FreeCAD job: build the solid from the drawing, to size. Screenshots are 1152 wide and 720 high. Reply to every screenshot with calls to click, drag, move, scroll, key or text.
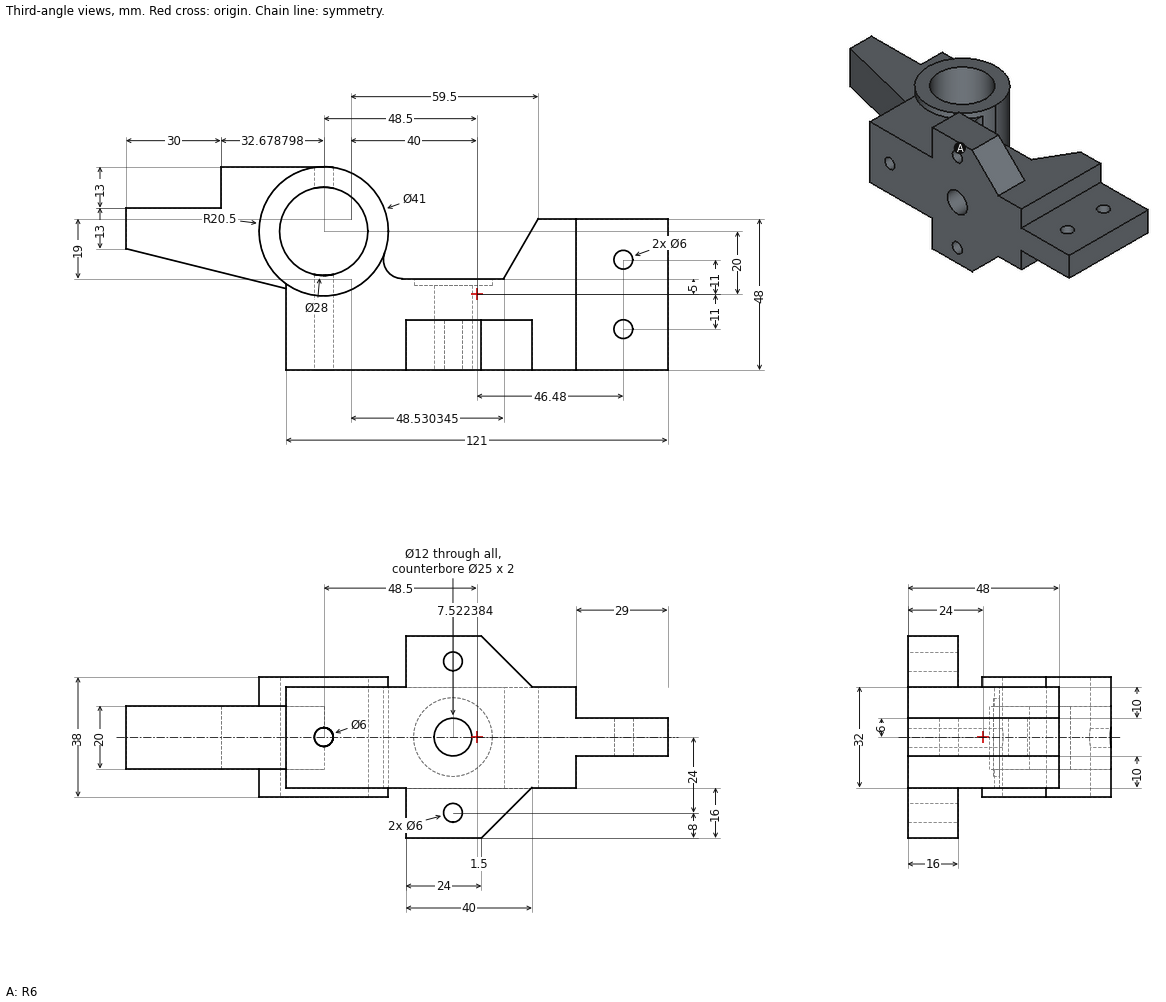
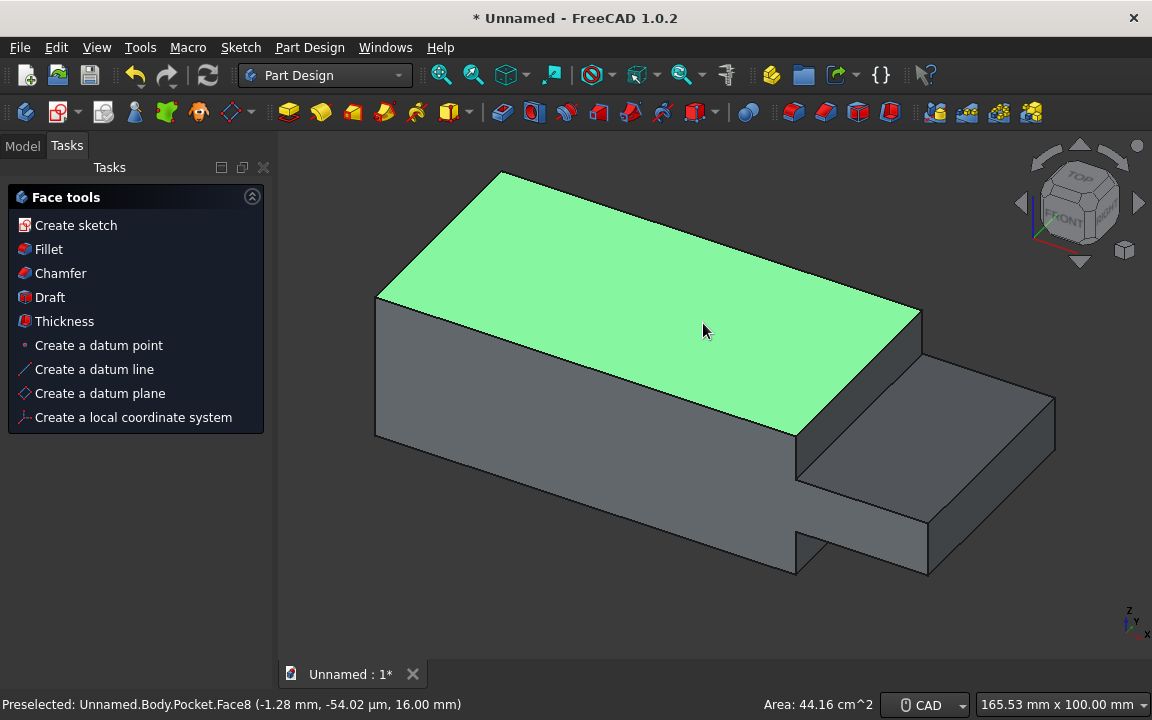
click(58, 112)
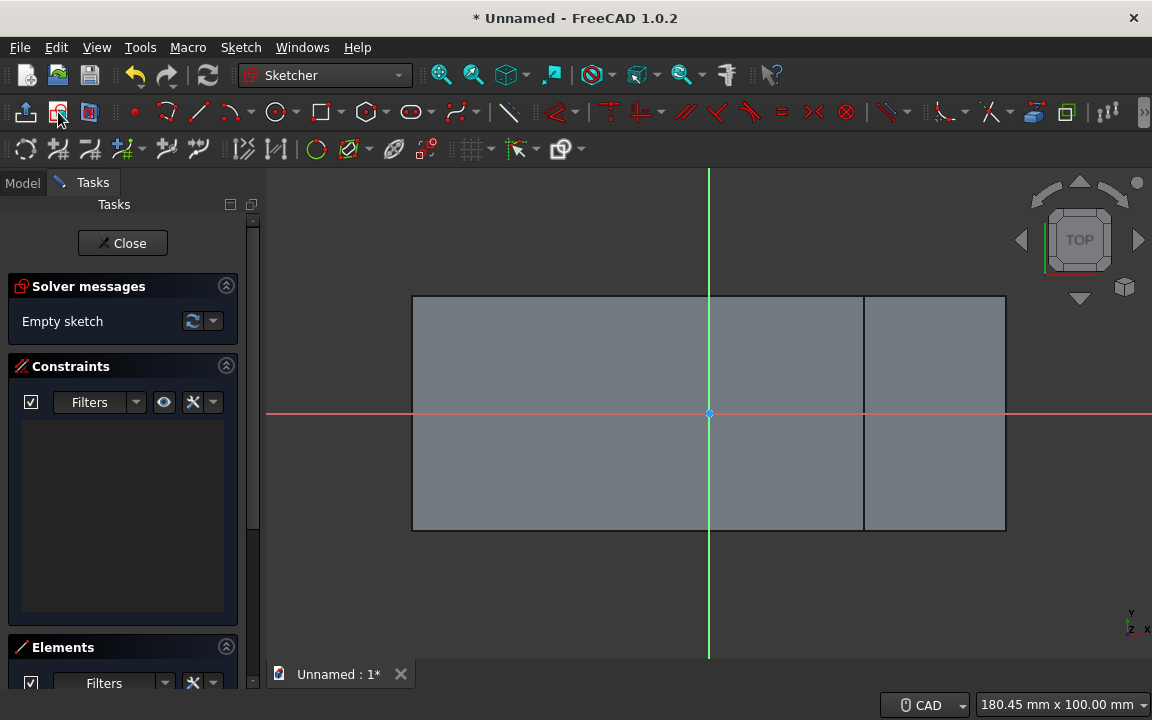
scroll(681, 283, up, 3)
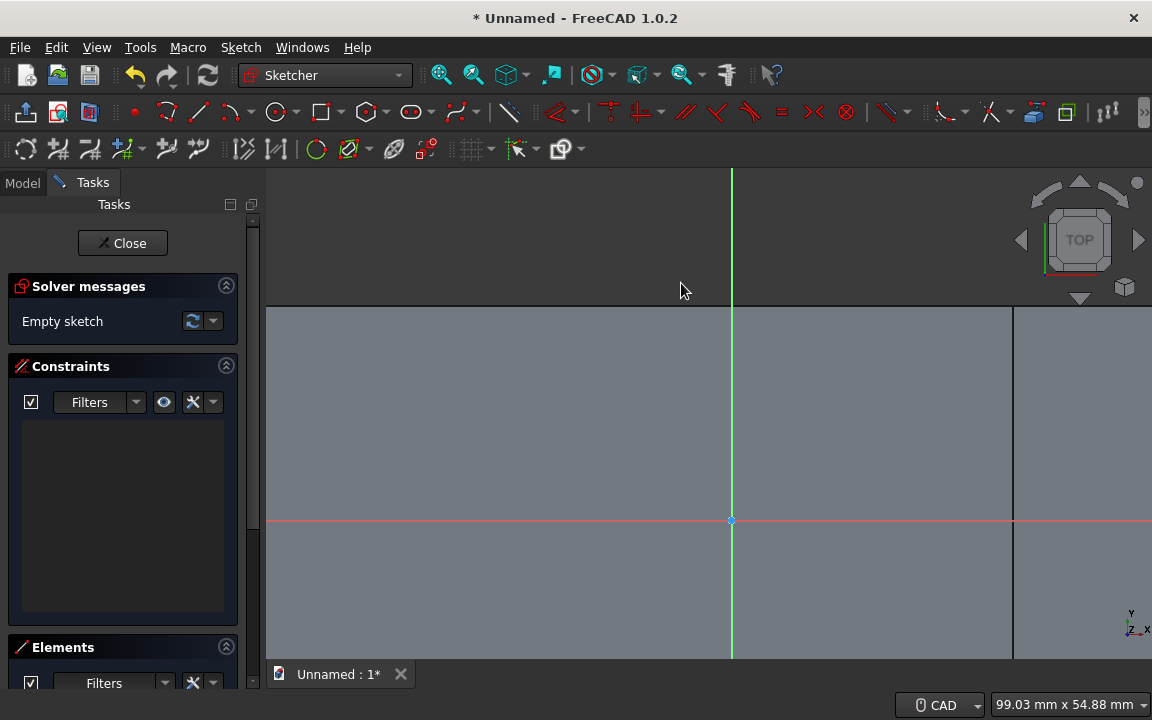
key(g)
key(m)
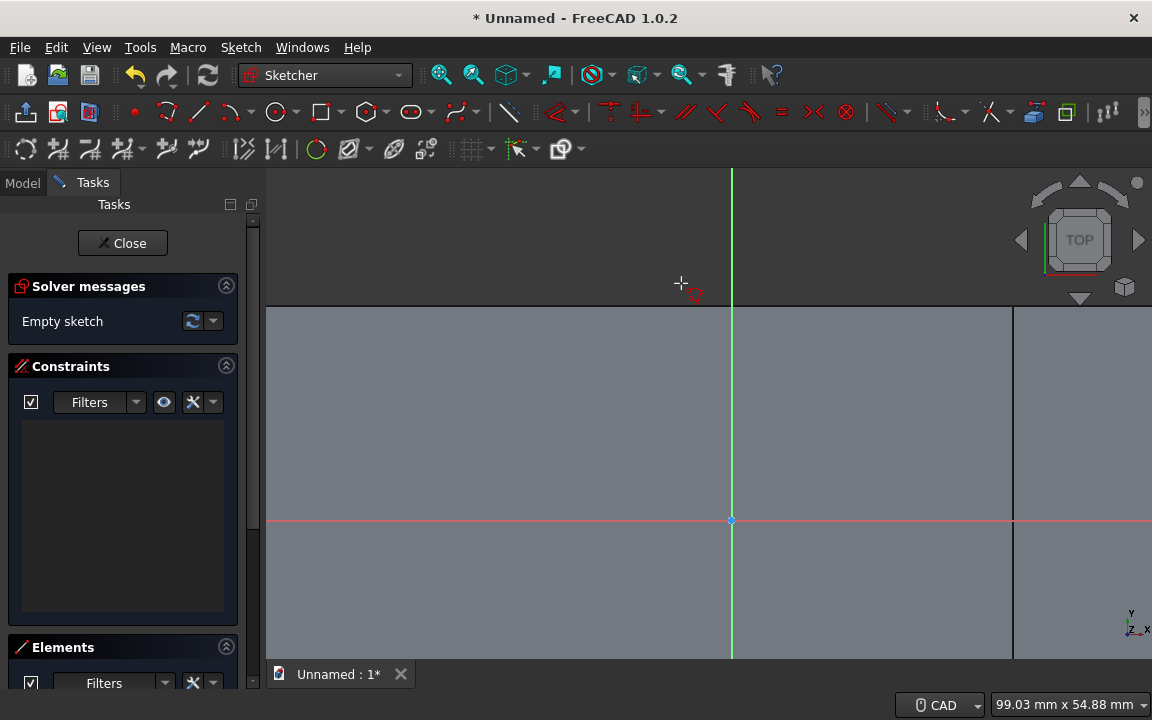
click(808, 476)
click(906, 306)
click(374, 306)
click(374, 476)
click(808, 477)
key(Escape)
key(Escape)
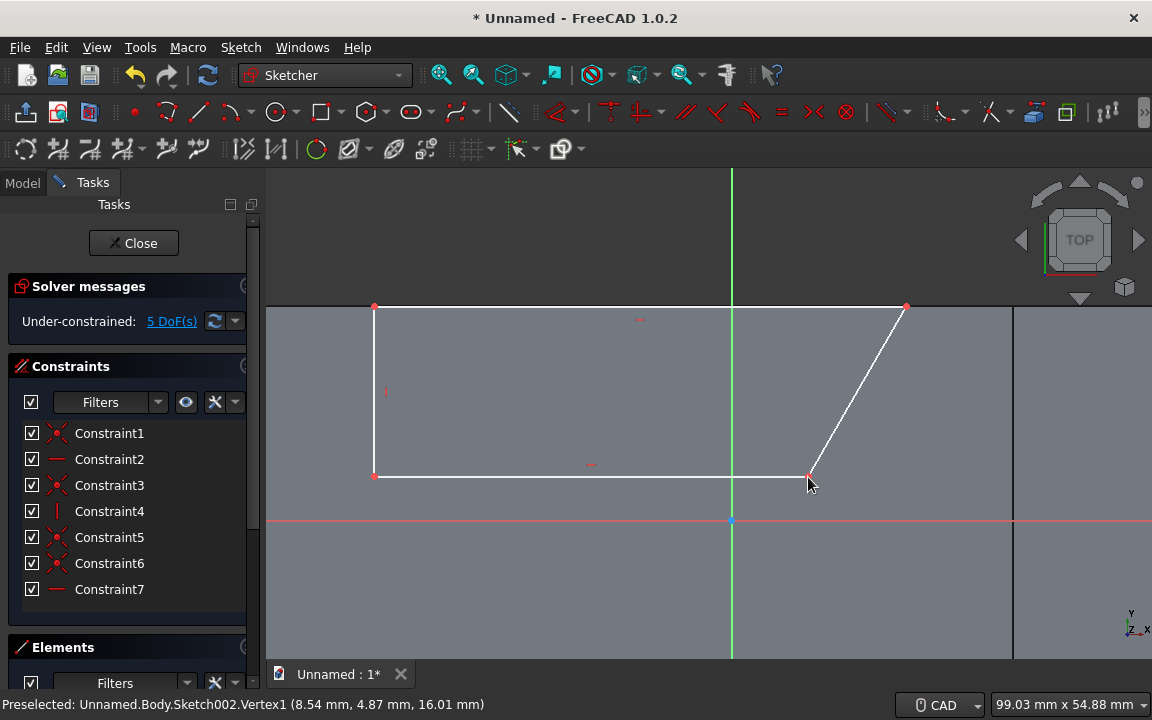
click(374, 358)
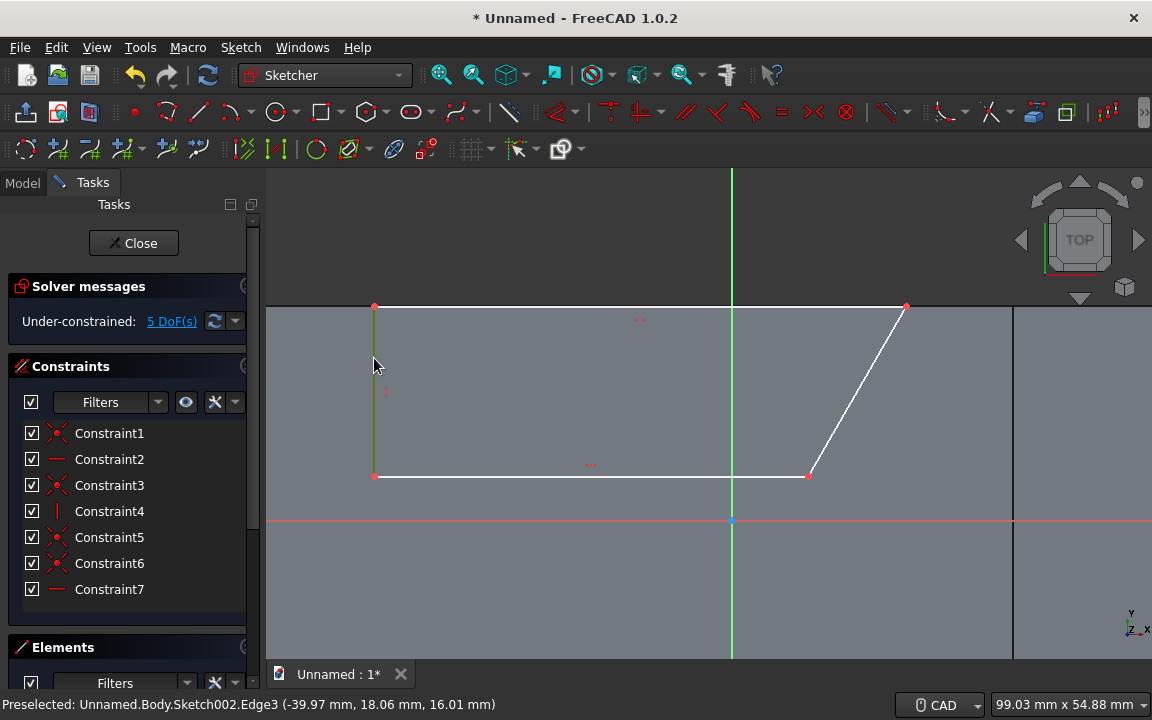
key(i)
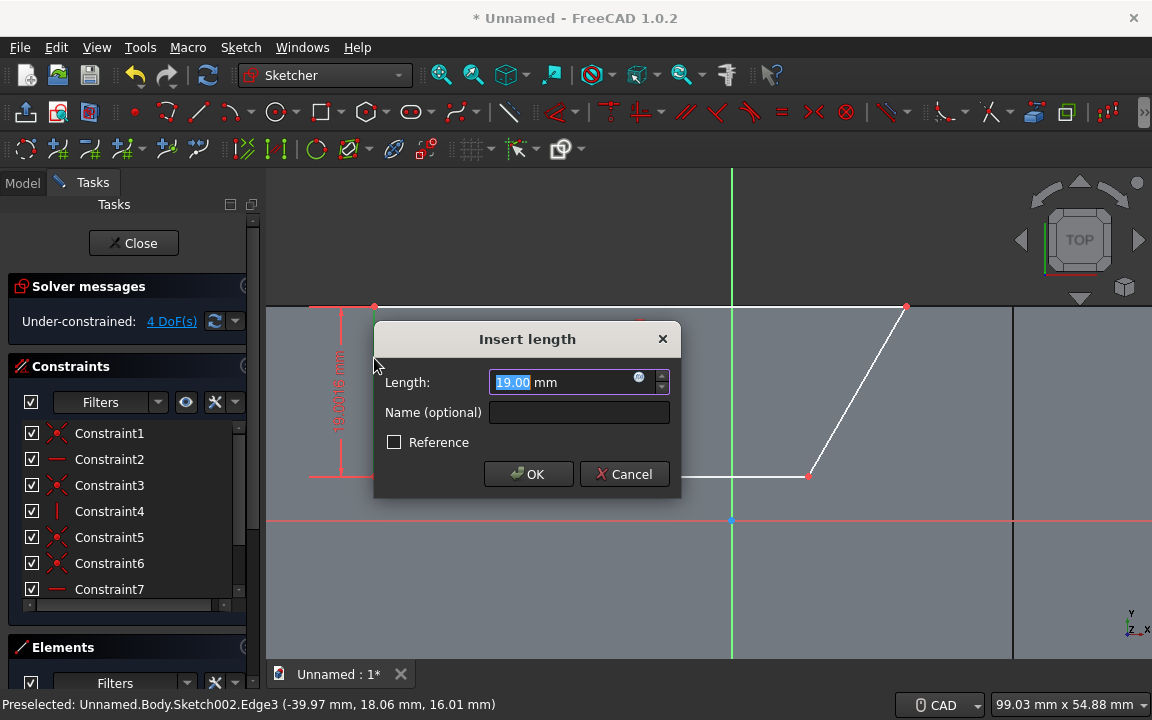
text(19)
key(Return)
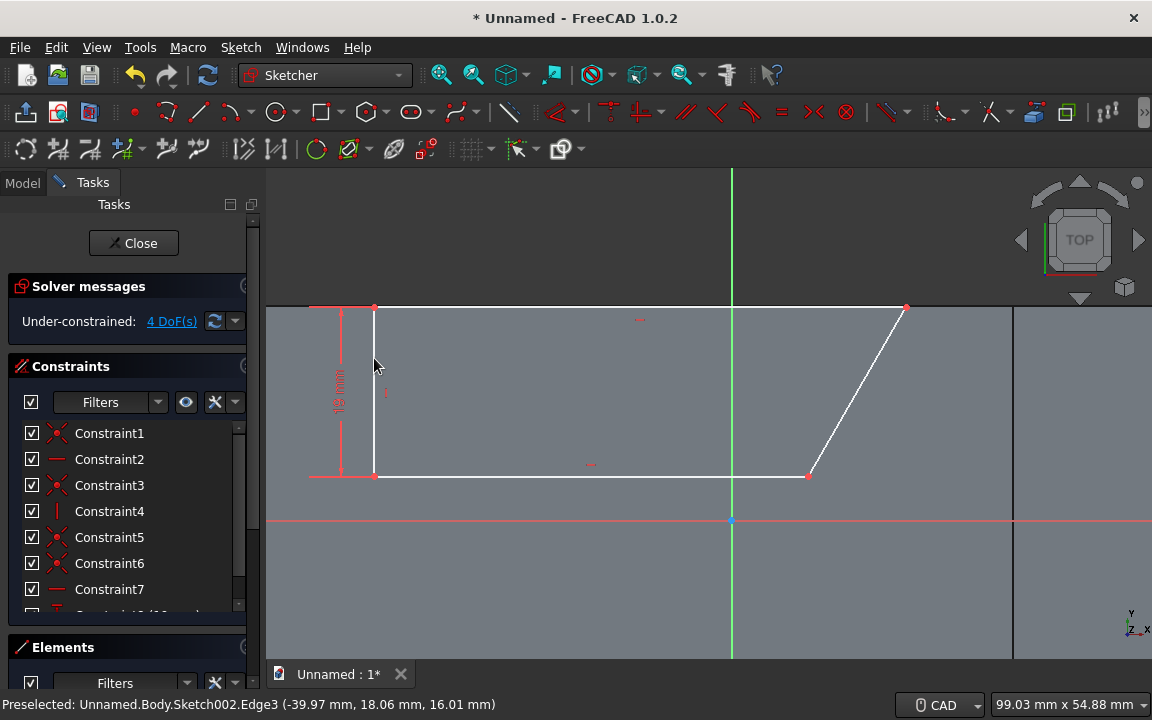
click(808, 477)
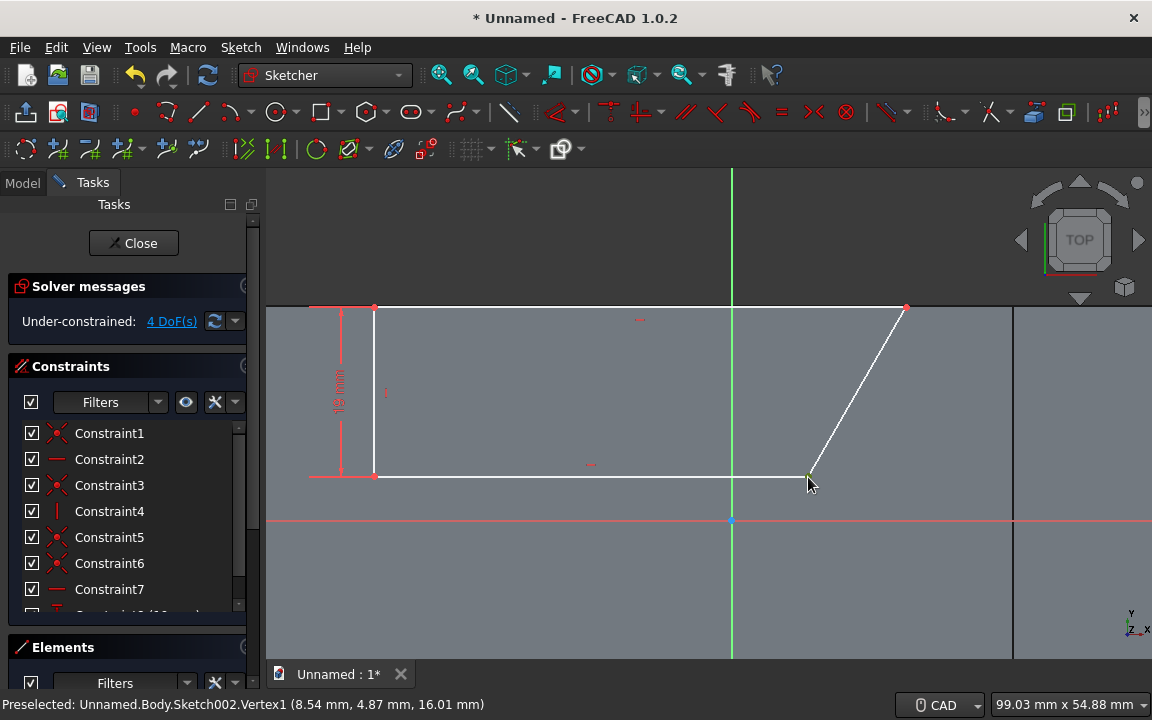
key(i)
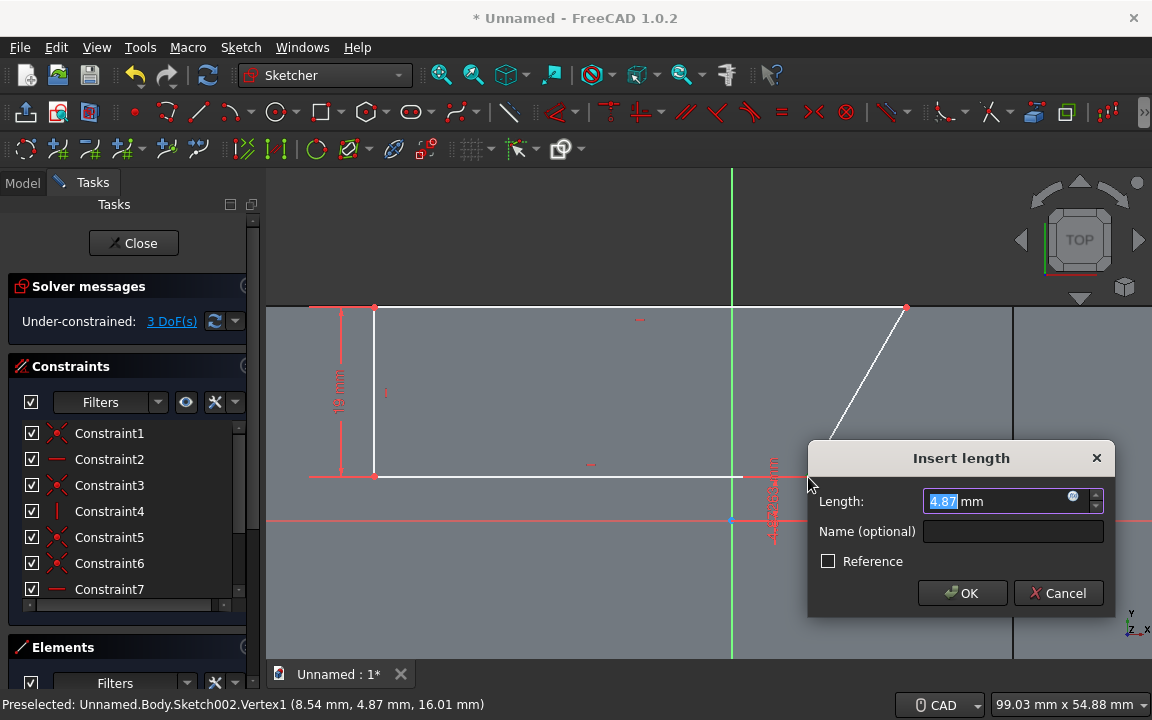
text(5)
key(Return)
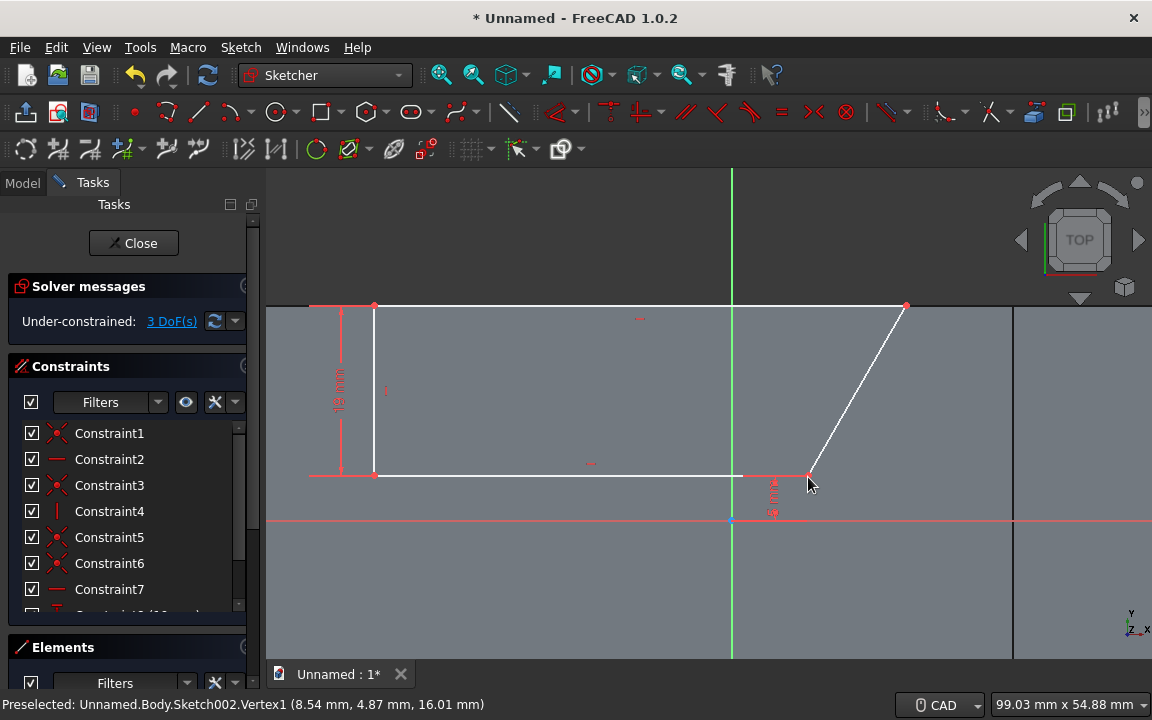
click(374, 306)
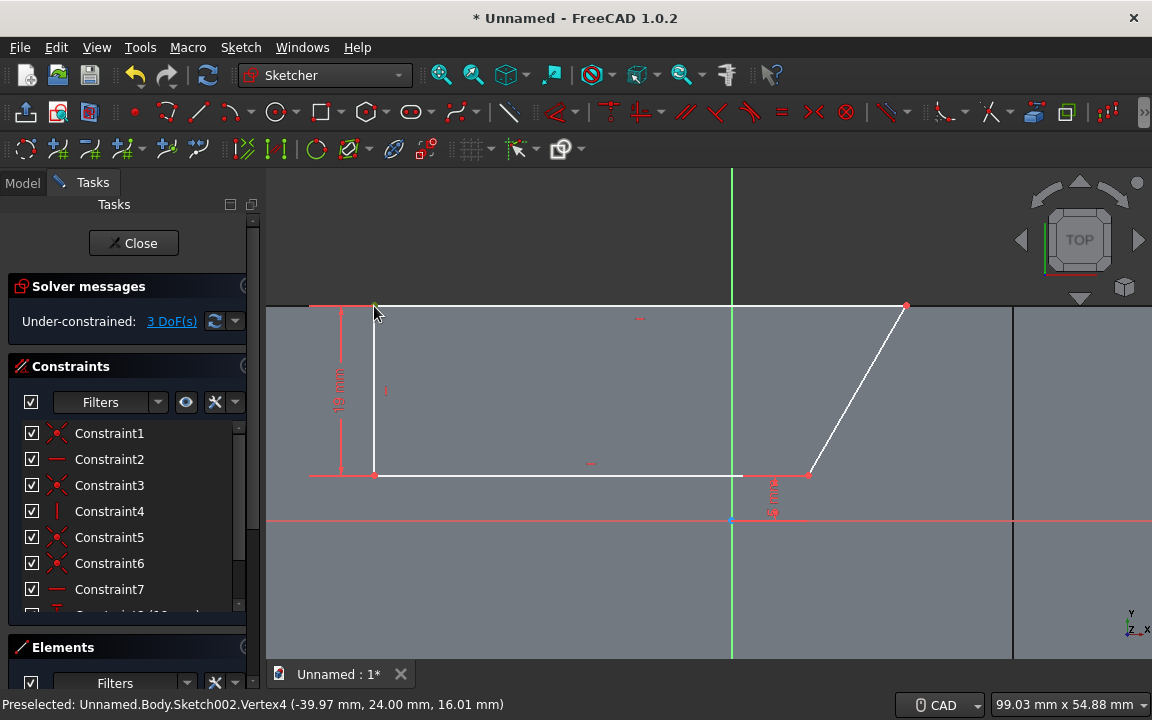
key(l)